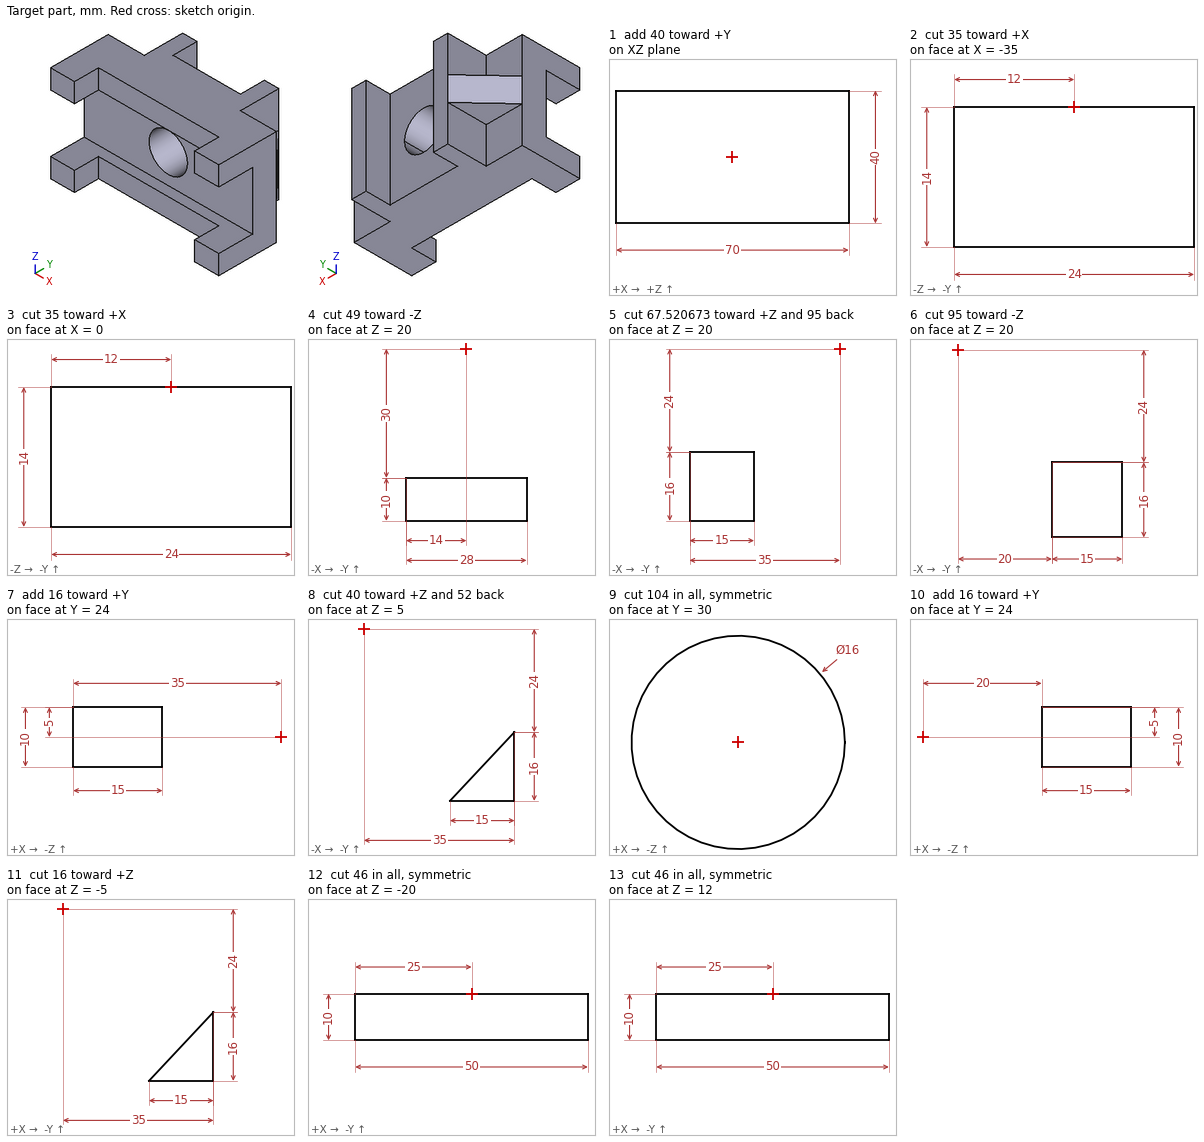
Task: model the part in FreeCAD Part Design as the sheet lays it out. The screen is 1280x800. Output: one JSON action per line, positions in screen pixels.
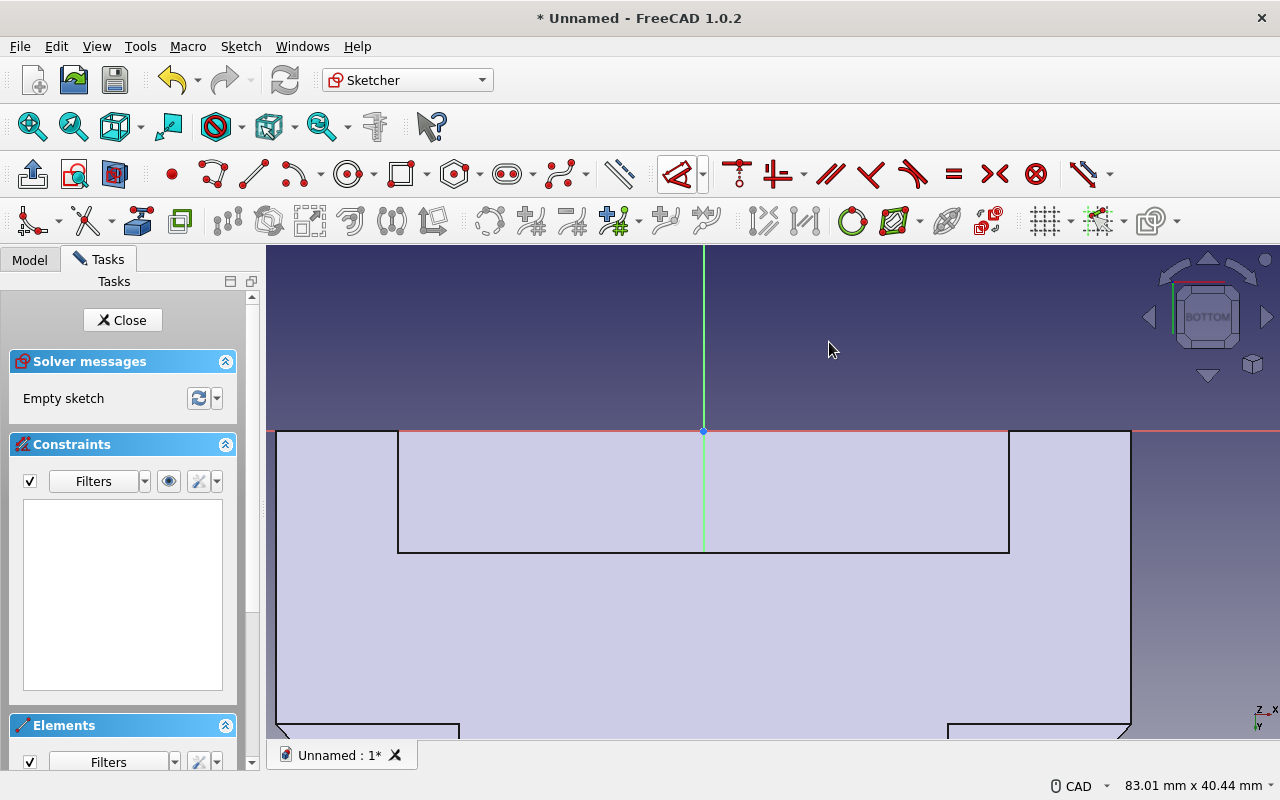
{"action": "left_click", "coordinate": [400, 174]}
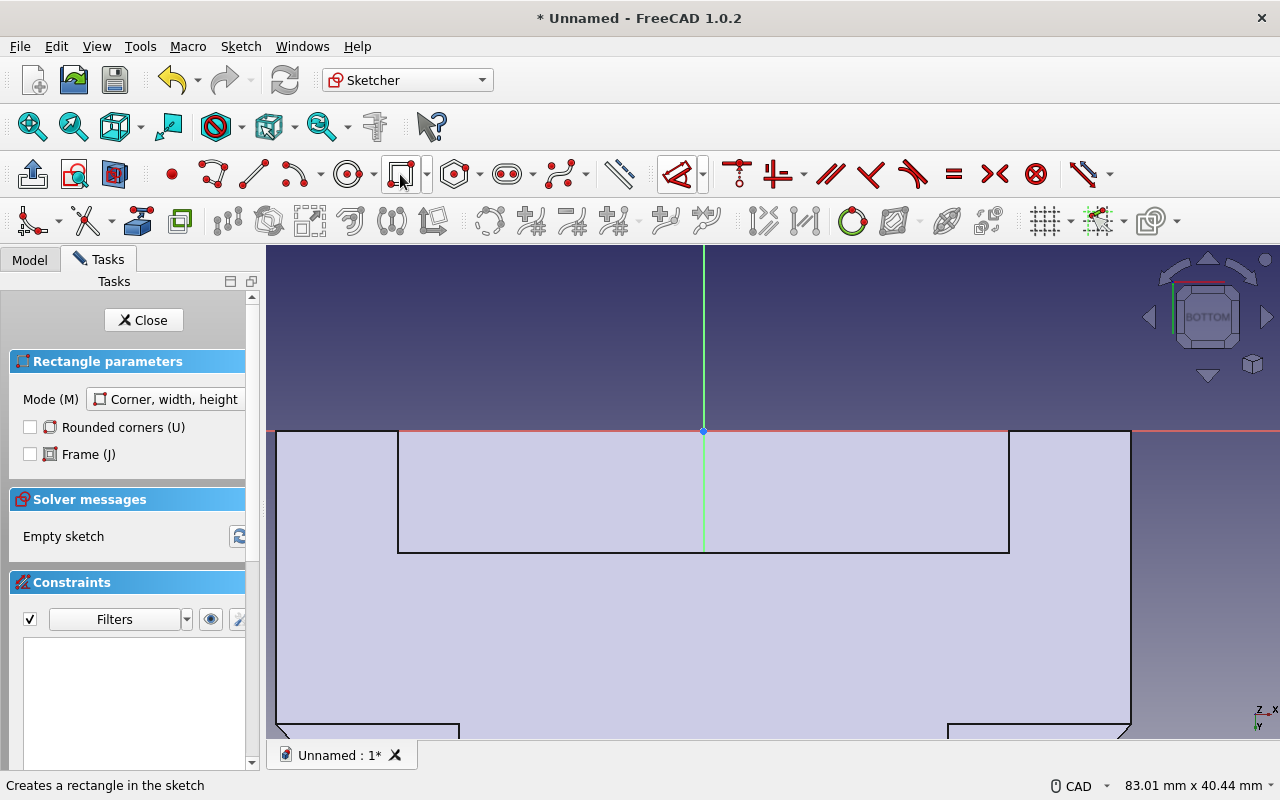
{"action": "left_click", "coordinate": [398, 431]}
{"action": "left_click", "coordinate": [1009, 553]}
{"action": "key", "text": "Escape"}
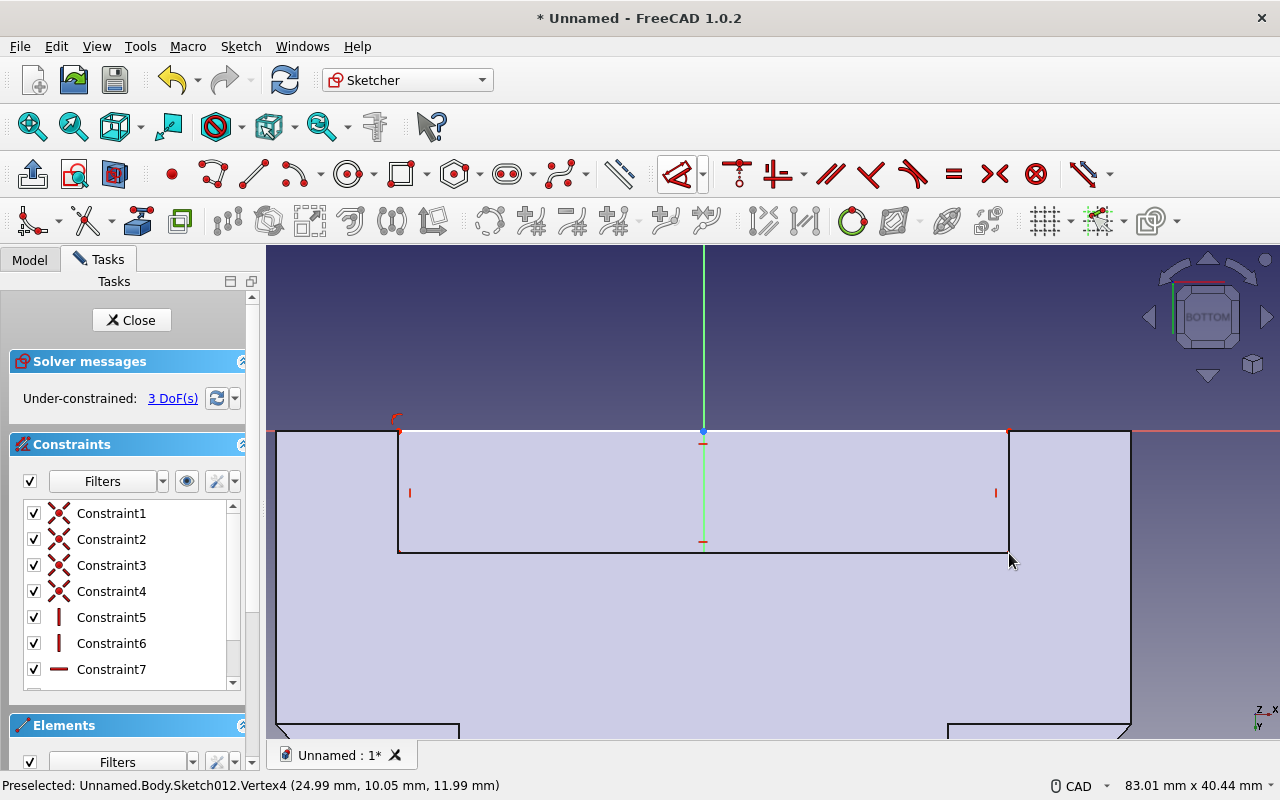
{"action": "left_click", "coordinate": [398, 468]}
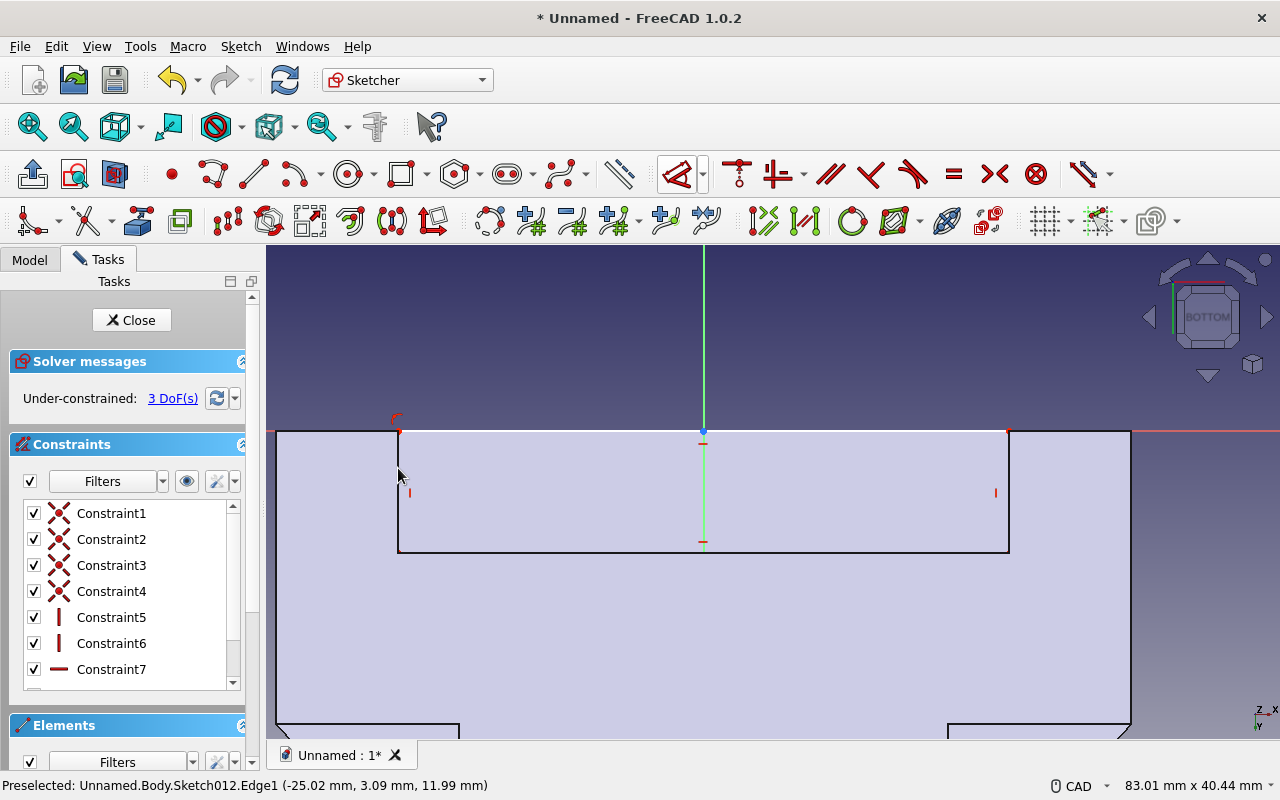
{"action": "key", "text": "i"}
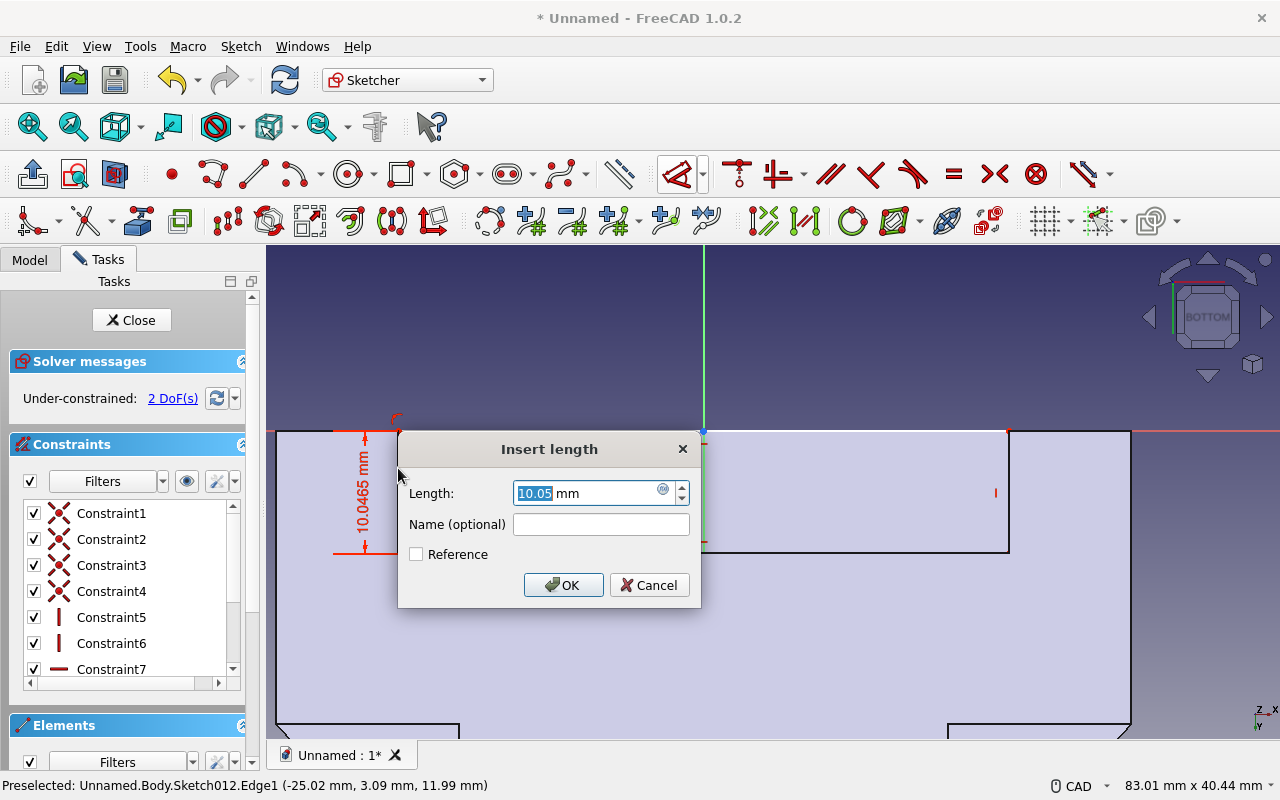
{"action": "type", "text": "10"}
{"action": "key", "text": "Return"}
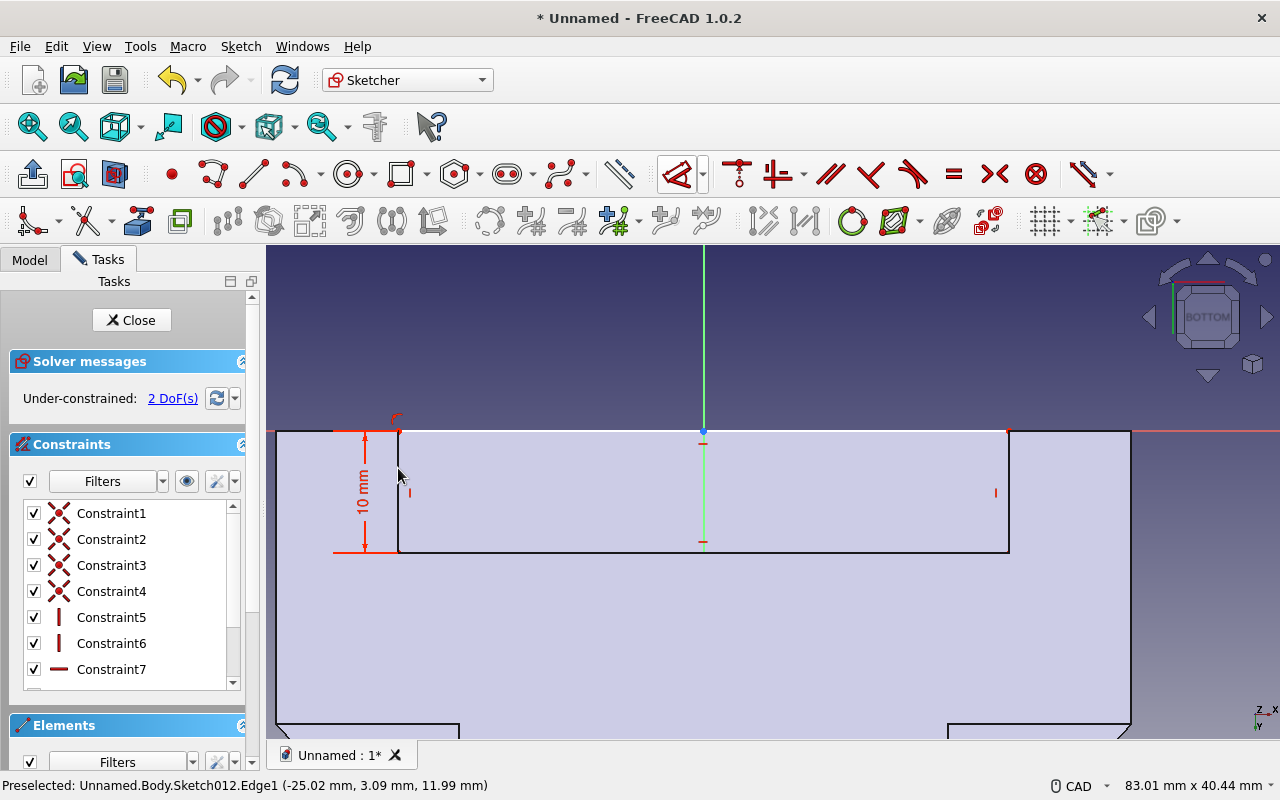
{"action": "left_click", "coordinate": [581, 553]}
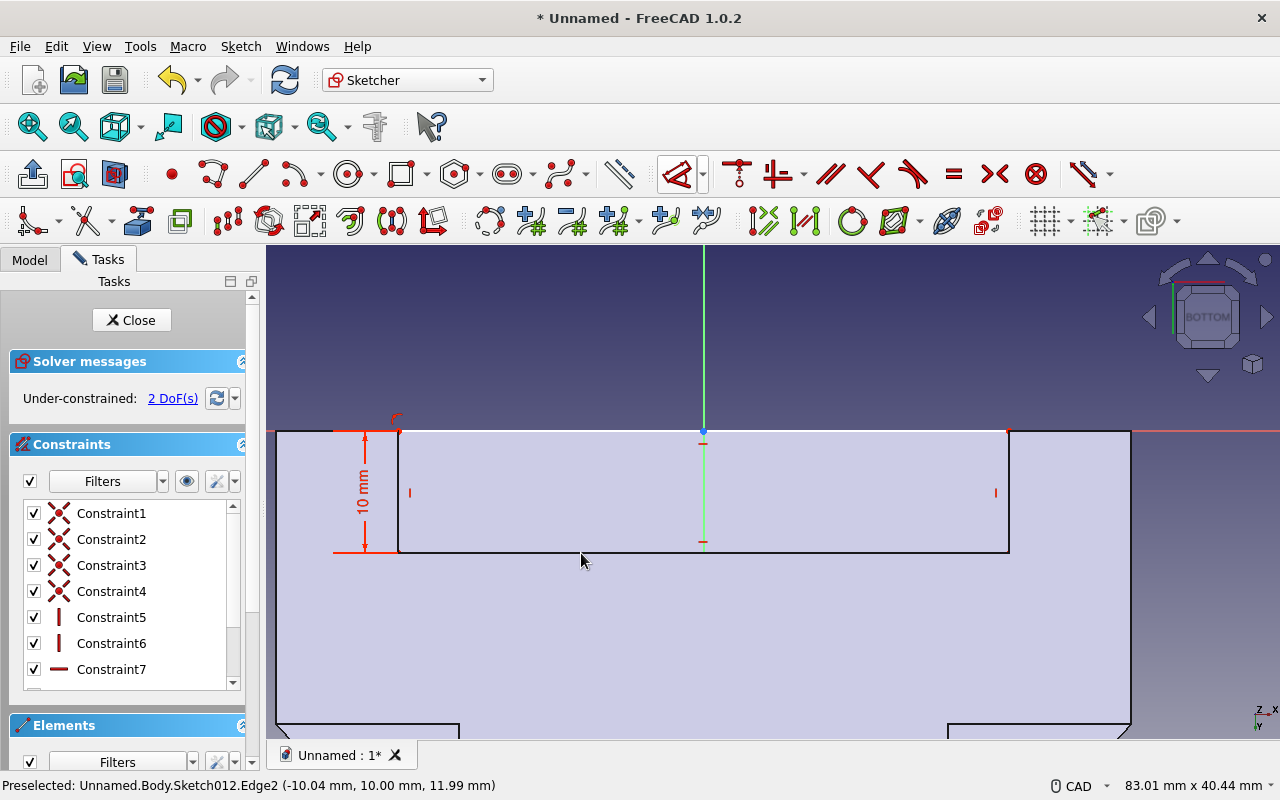
{"action": "key", "text": "l"}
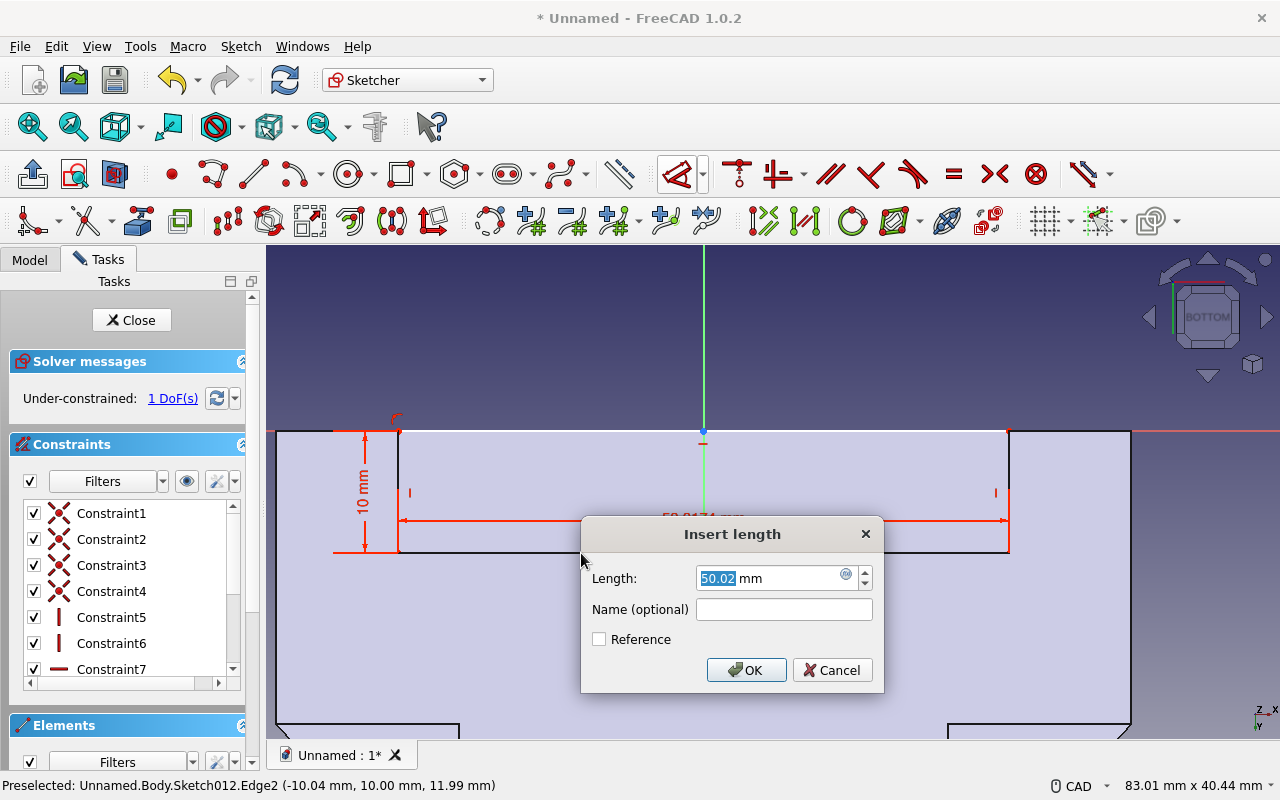
{"action": "type", "text": "50"}
{"action": "key", "text": "Return"}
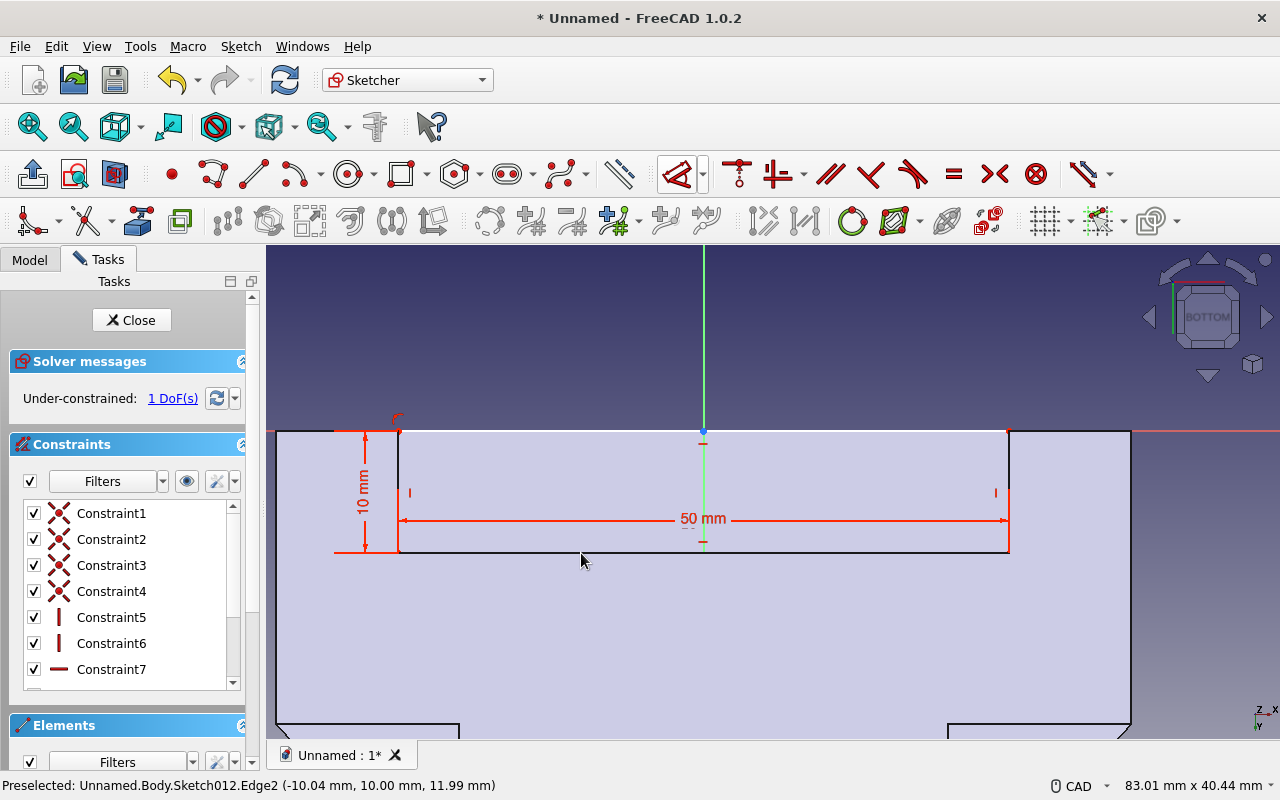
{"action": "left_click", "coordinate": [398, 431]}